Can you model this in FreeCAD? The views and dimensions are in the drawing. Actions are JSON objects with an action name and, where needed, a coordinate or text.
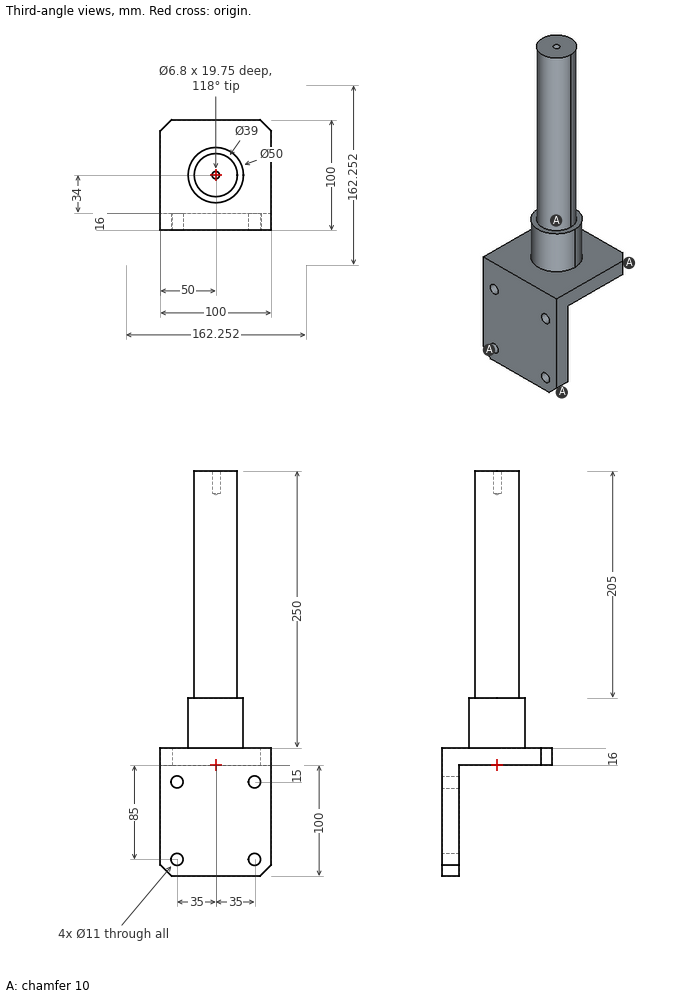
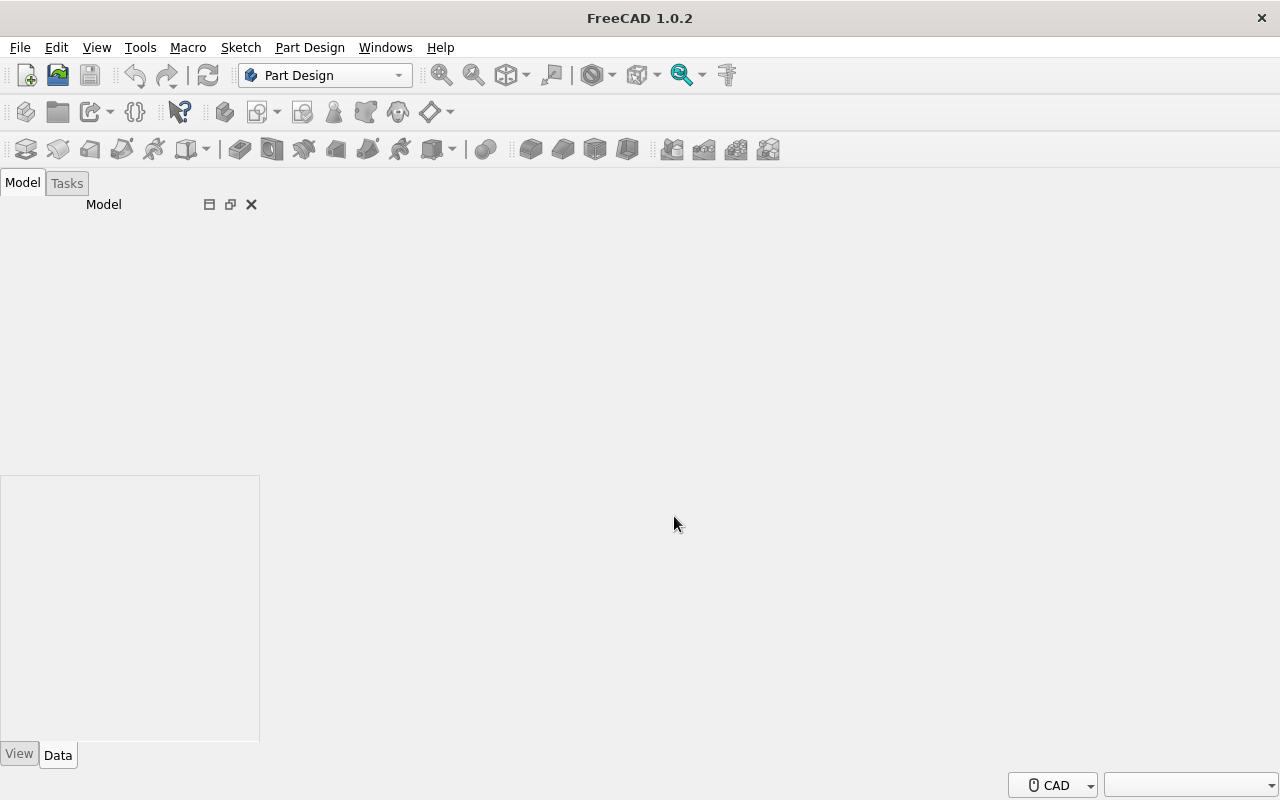
{"action": "left_click", "coordinate": [26, 76]}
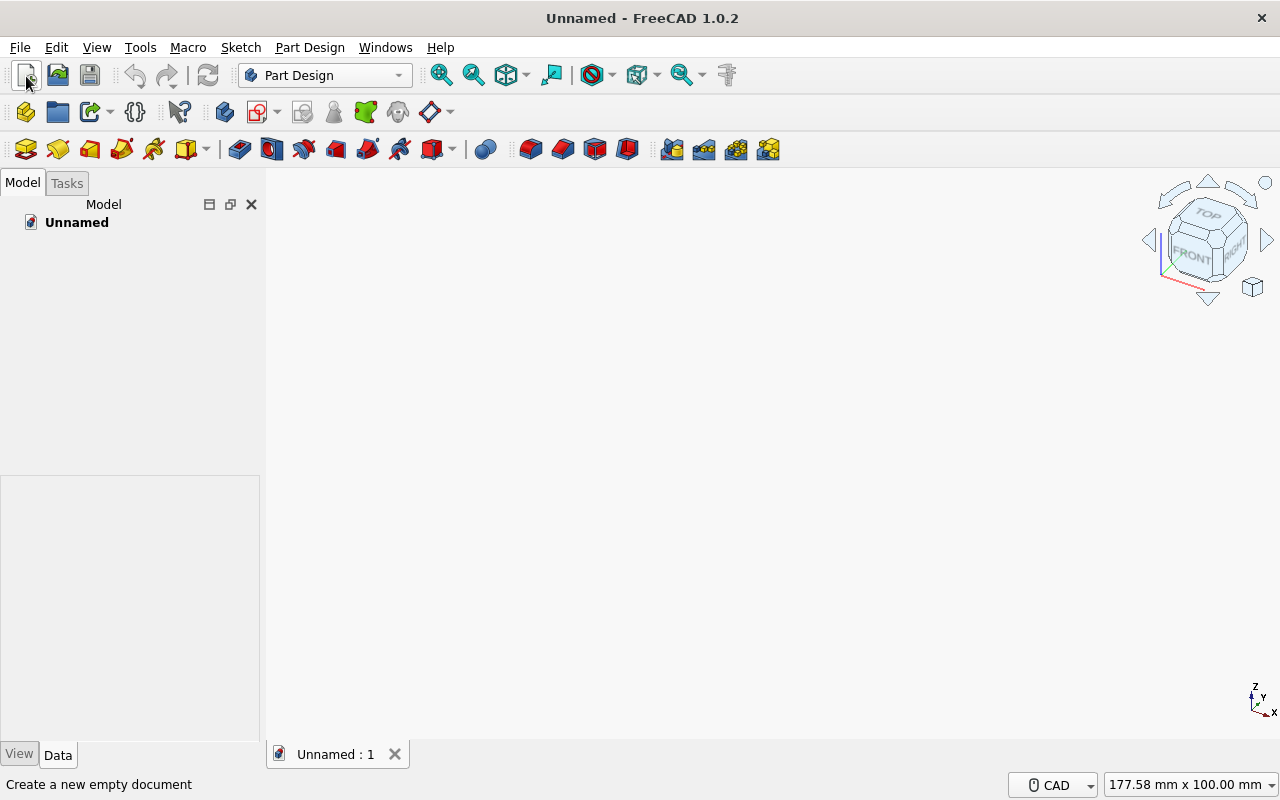
{"action": "left_click", "coordinate": [258, 112]}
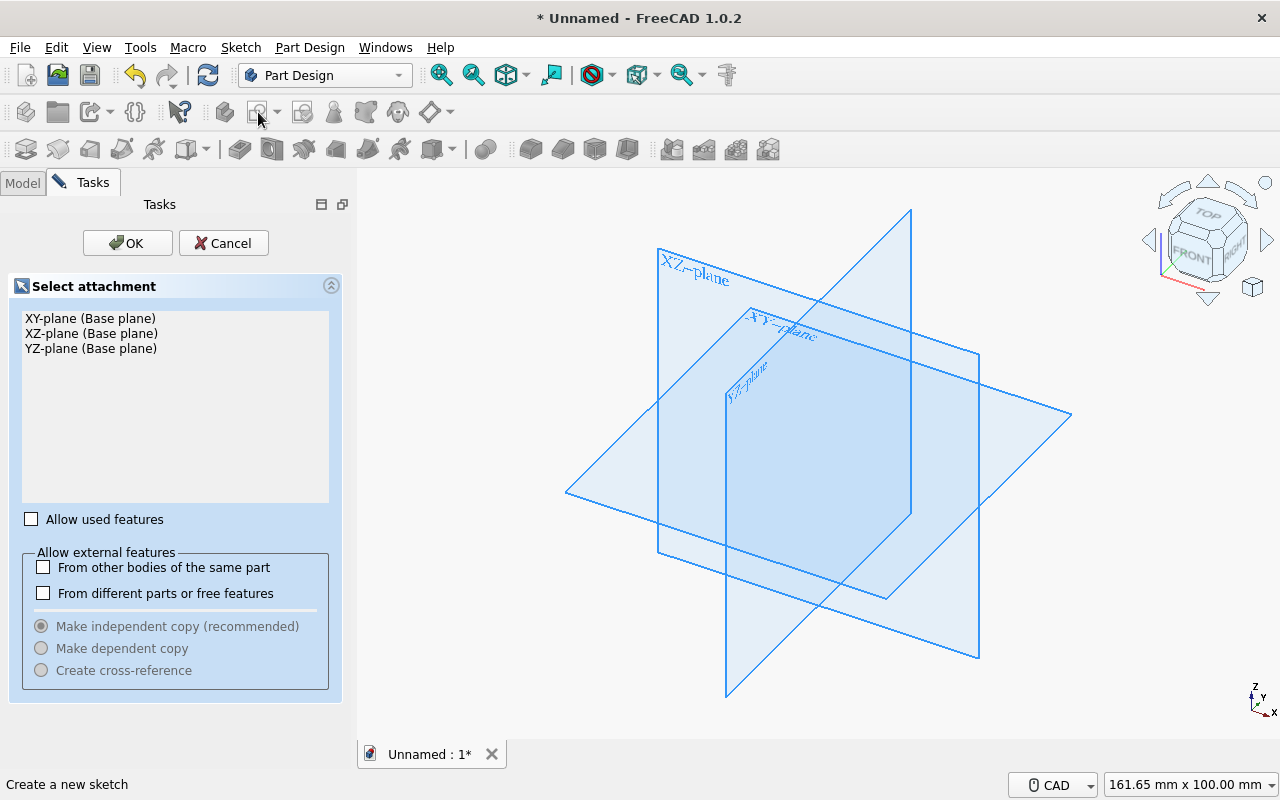
{"action": "left_click", "coordinate": [82, 318]}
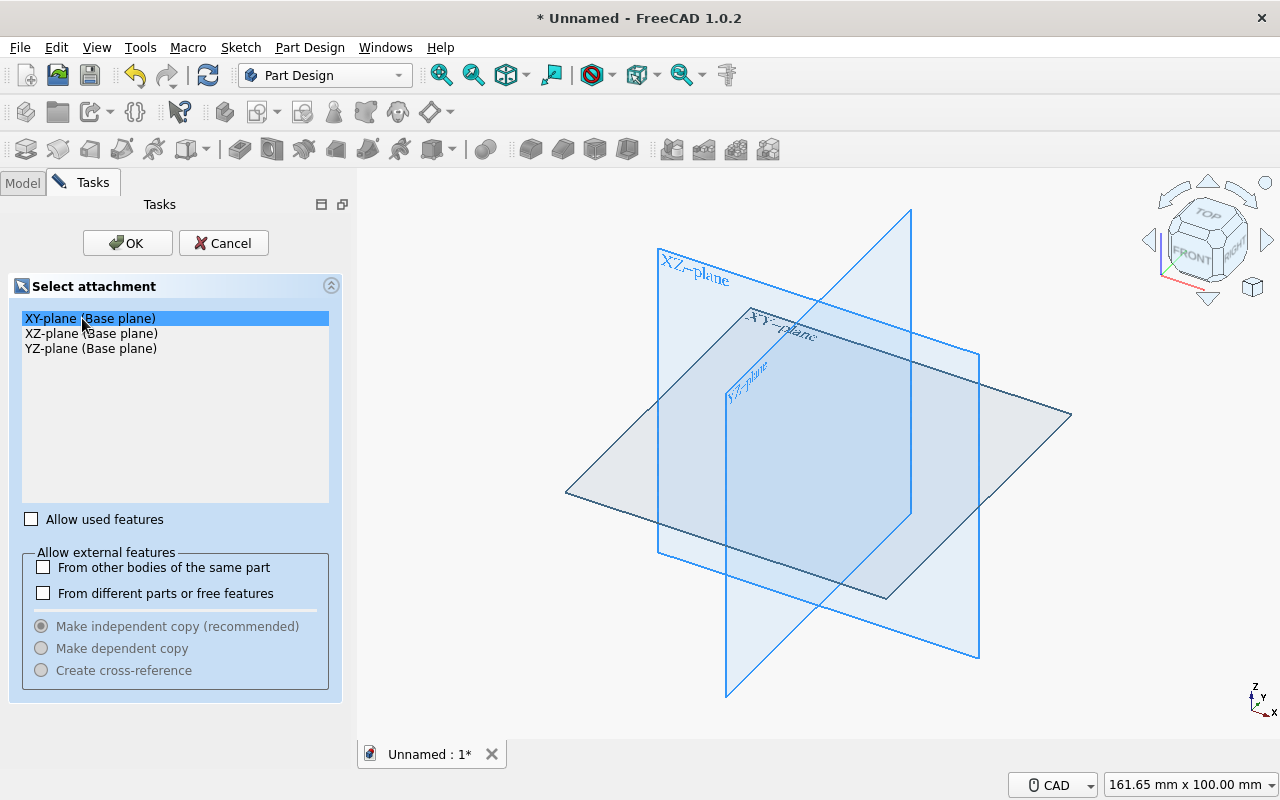
{"action": "left_click", "coordinate": [128, 243]}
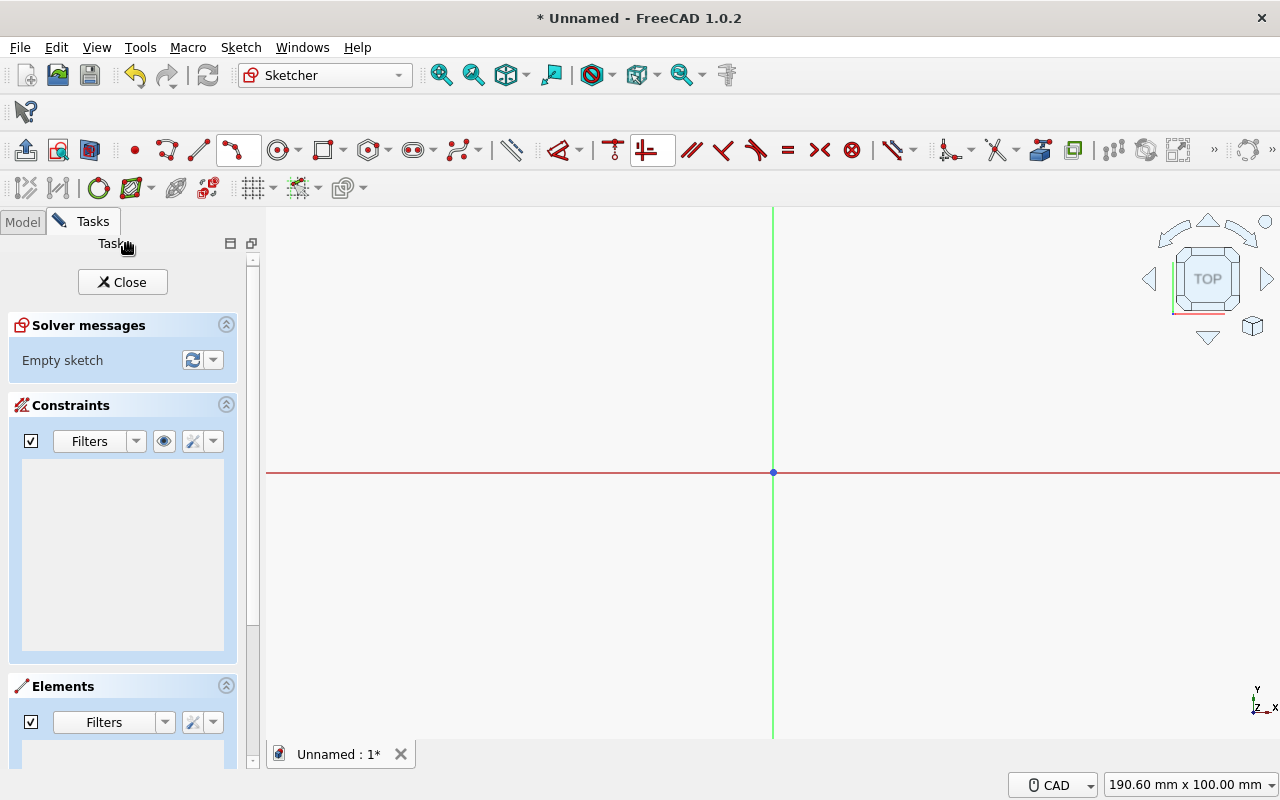
{"action": "scroll", "coordinate": [565, 473], "scroll_direction": "down", "scroll_amount": 2}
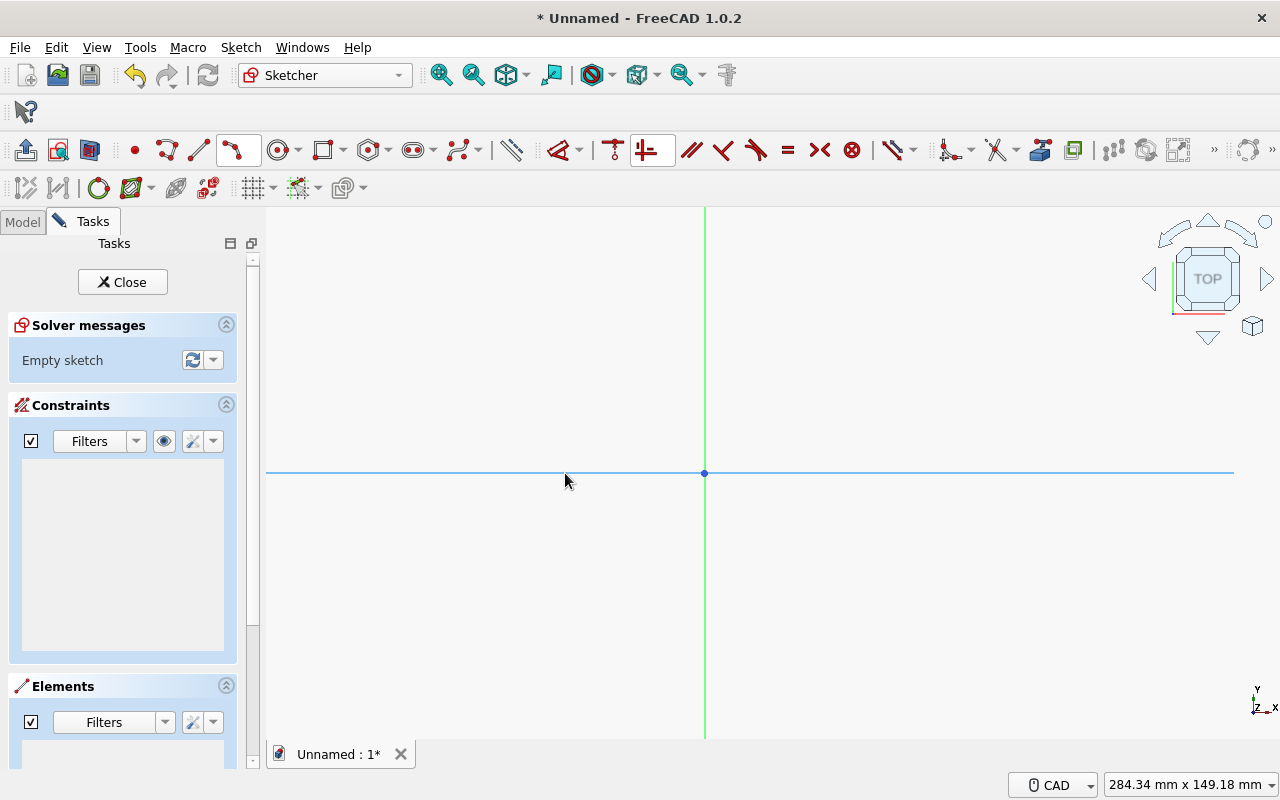
{"action": "key", "text": "g v"}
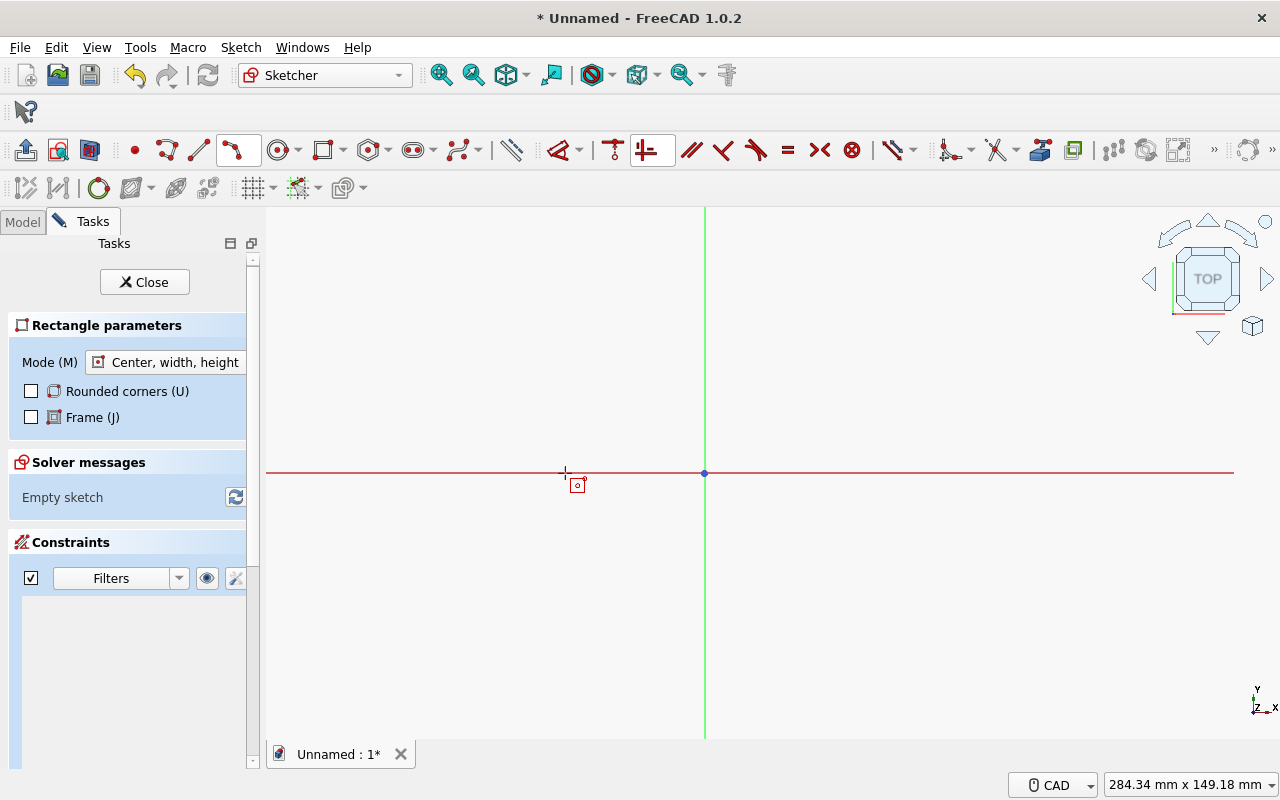
{"action": "left_click", "coordinate": [705, 473]}
{"action": "left_click", "coordinate": [883, 295]}
{"action": "key", "text": "Escape"}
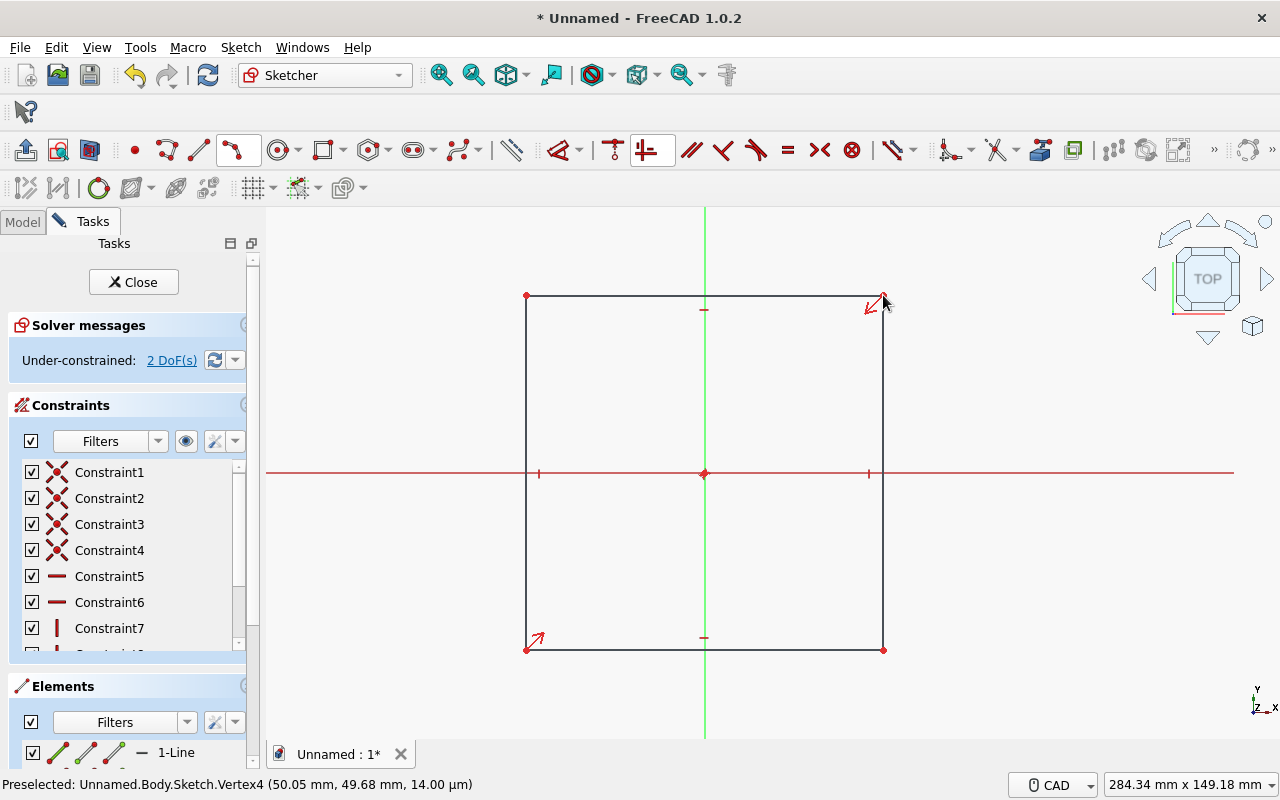
{"action": "key", "text": "d"}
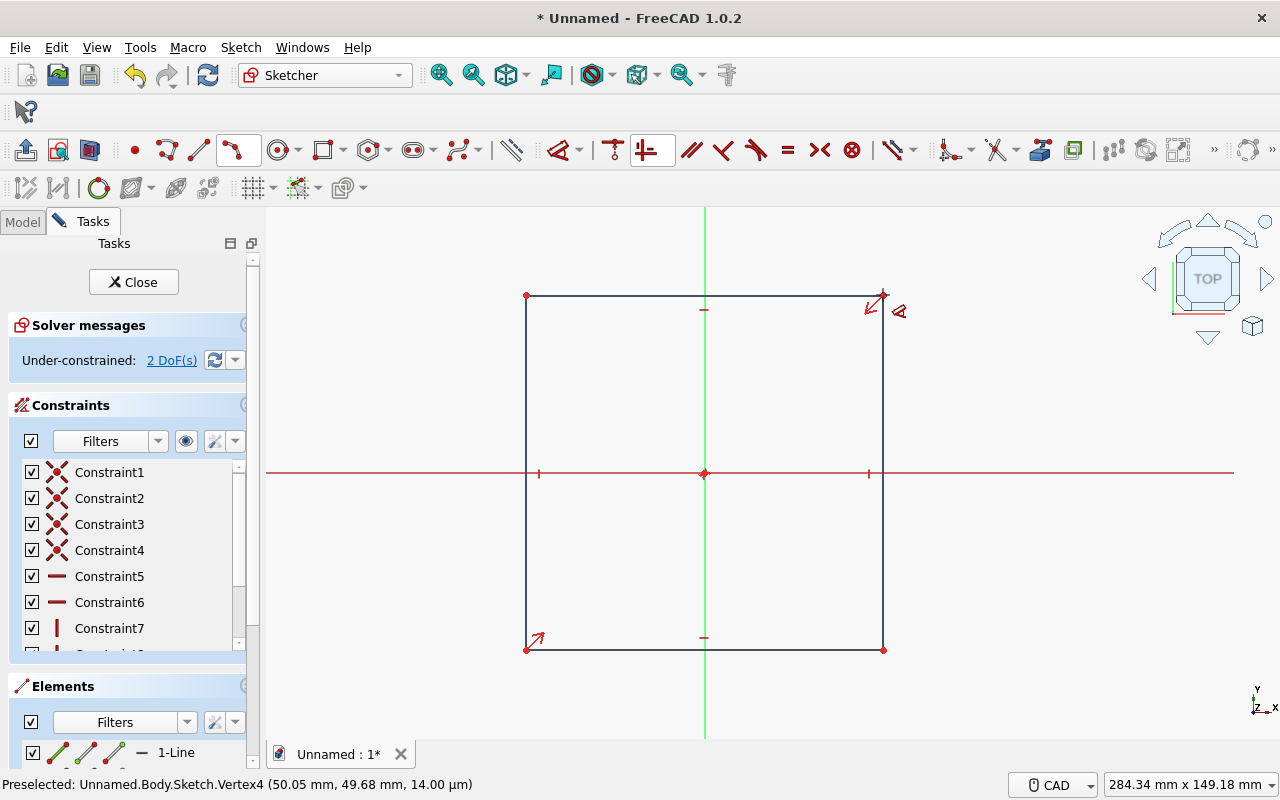
{"action": "left_click", "coordinate": [633, 650]}
{"action": "left_click", "coordinate": [622, 684]}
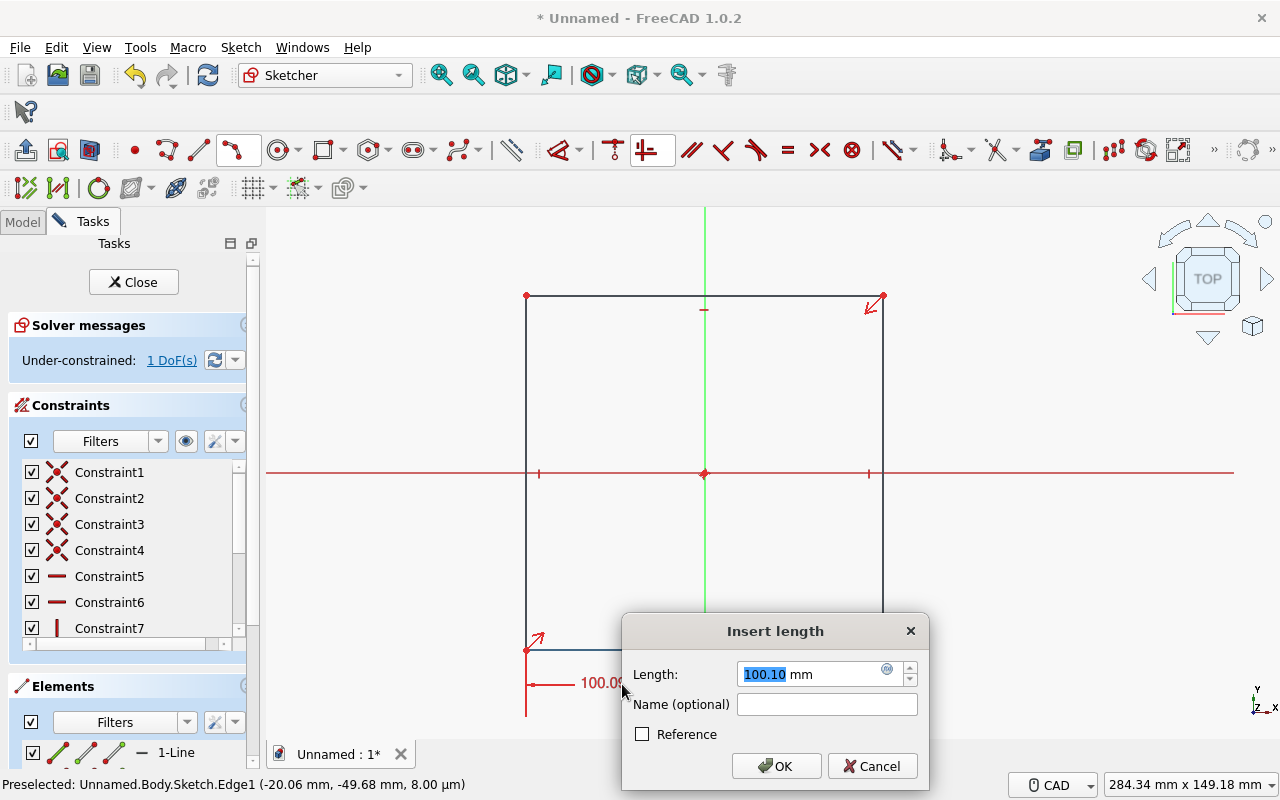
{"action": "type", "text": "100"}
{"action": "key", "text": "Return"}